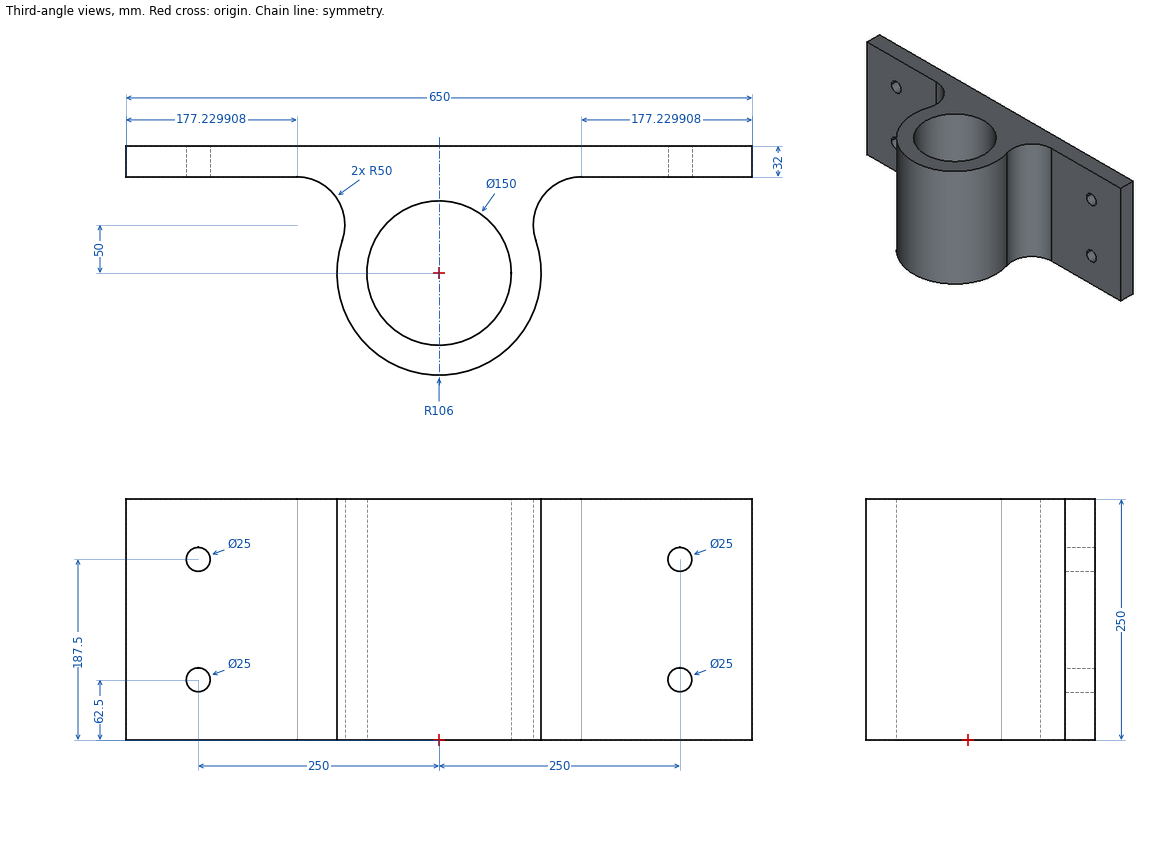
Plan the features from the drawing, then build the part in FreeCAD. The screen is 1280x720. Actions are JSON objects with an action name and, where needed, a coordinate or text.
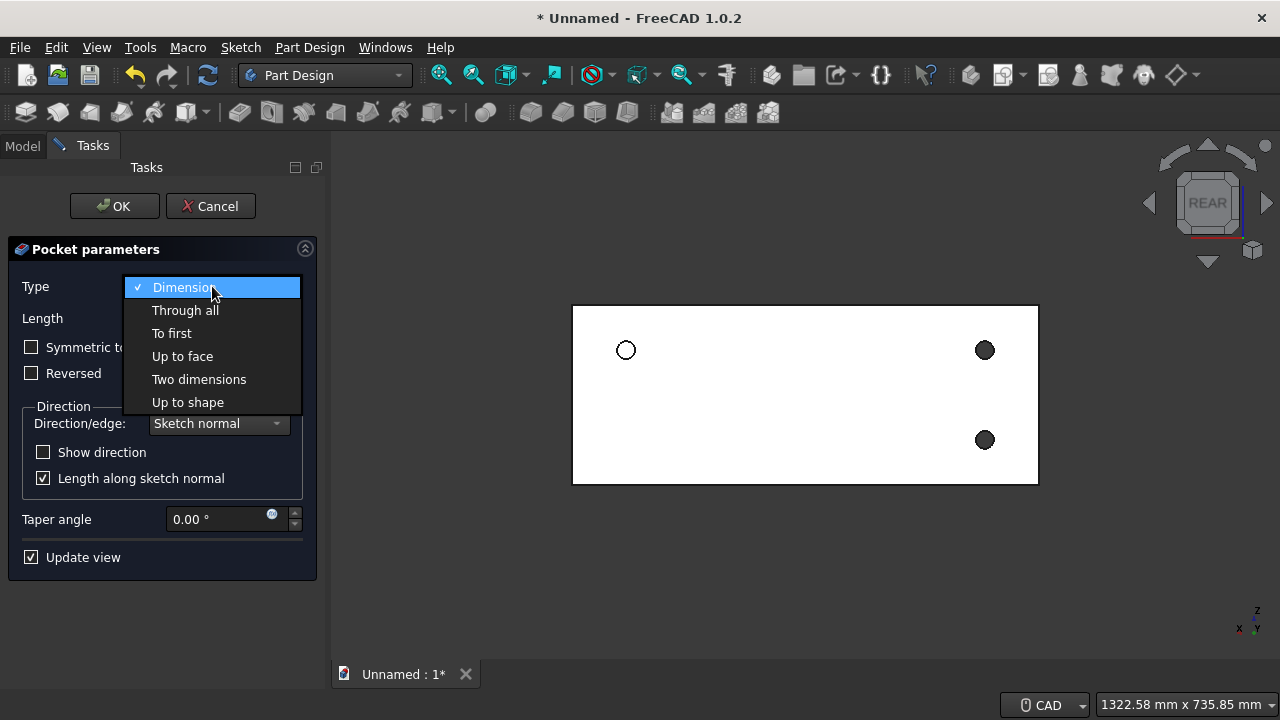
{"action": "left_click", "coordinate": [212, 334]}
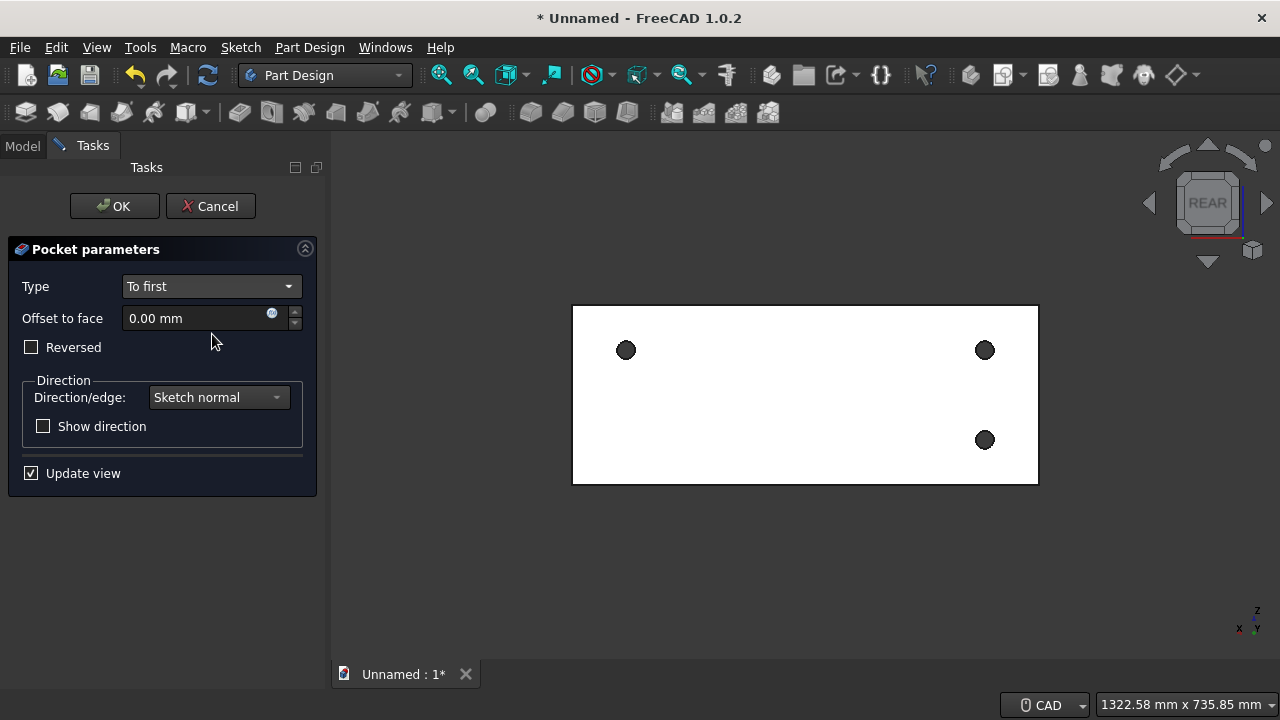
{"action": "left_click", "coordinate": [115, 206]}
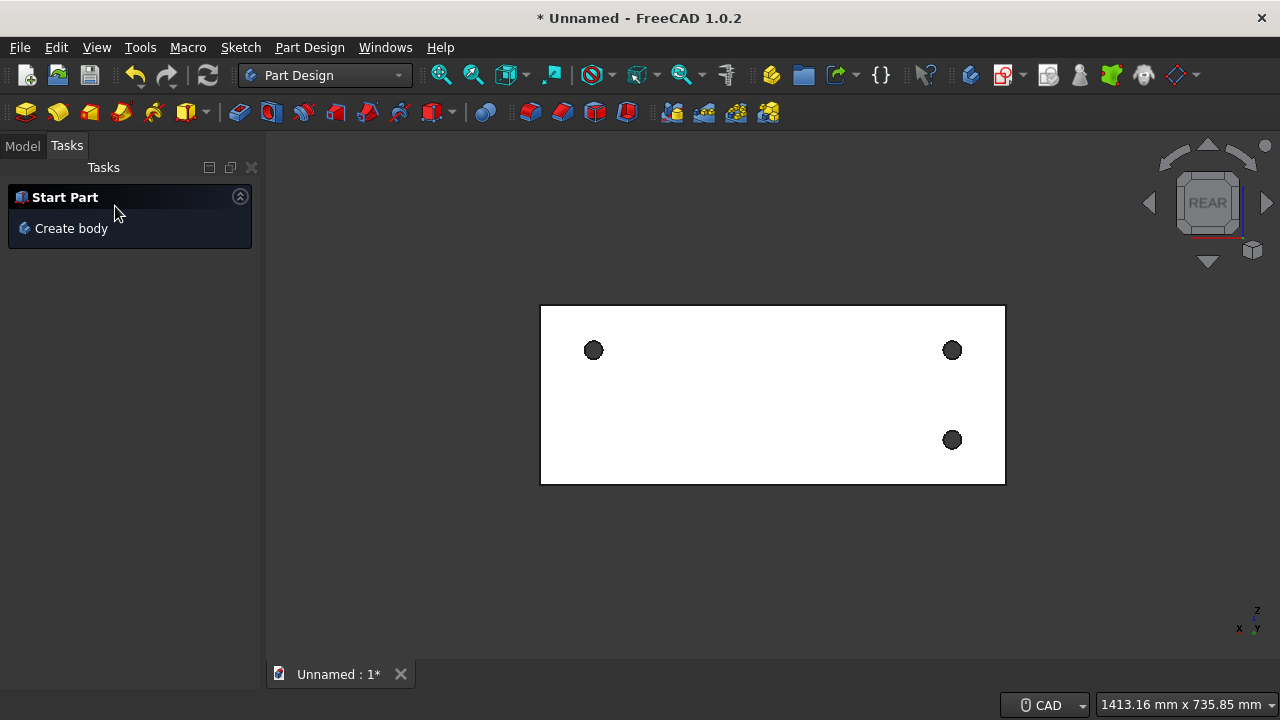
{"action": "left_click", "coordinate": [706, 394]}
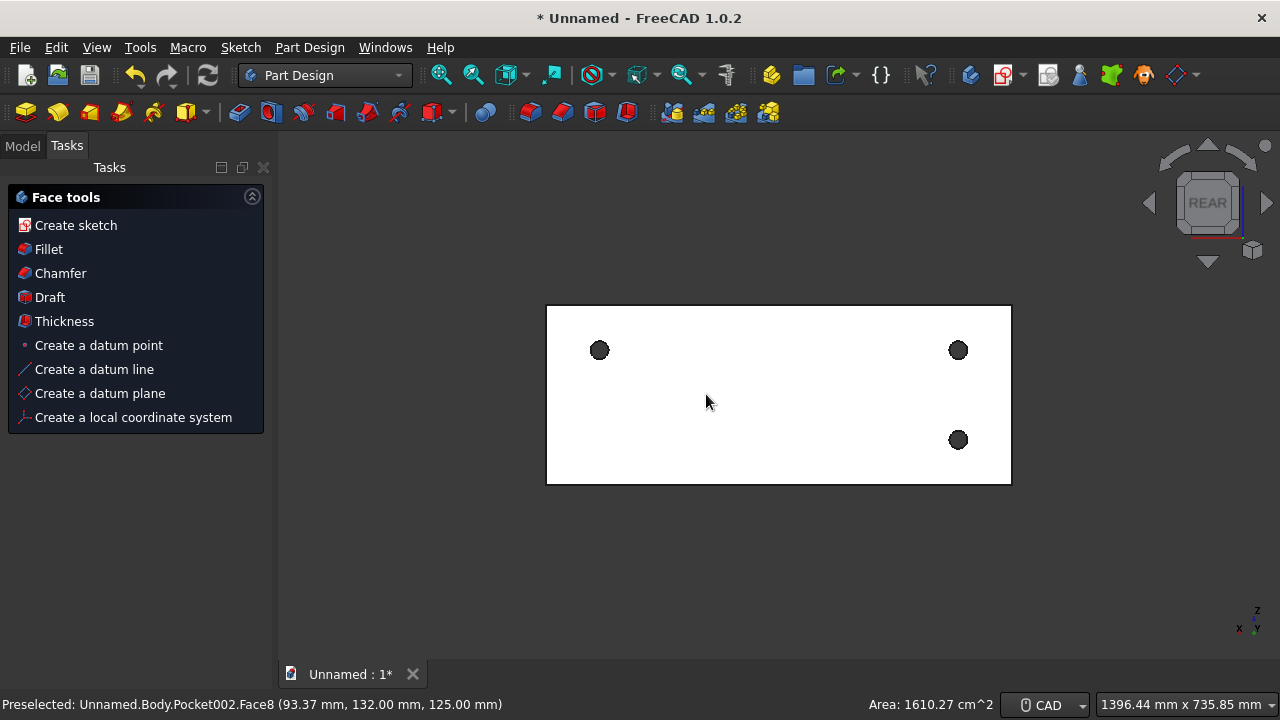
{"action": "left_click", "coordinate": [1004, 76]}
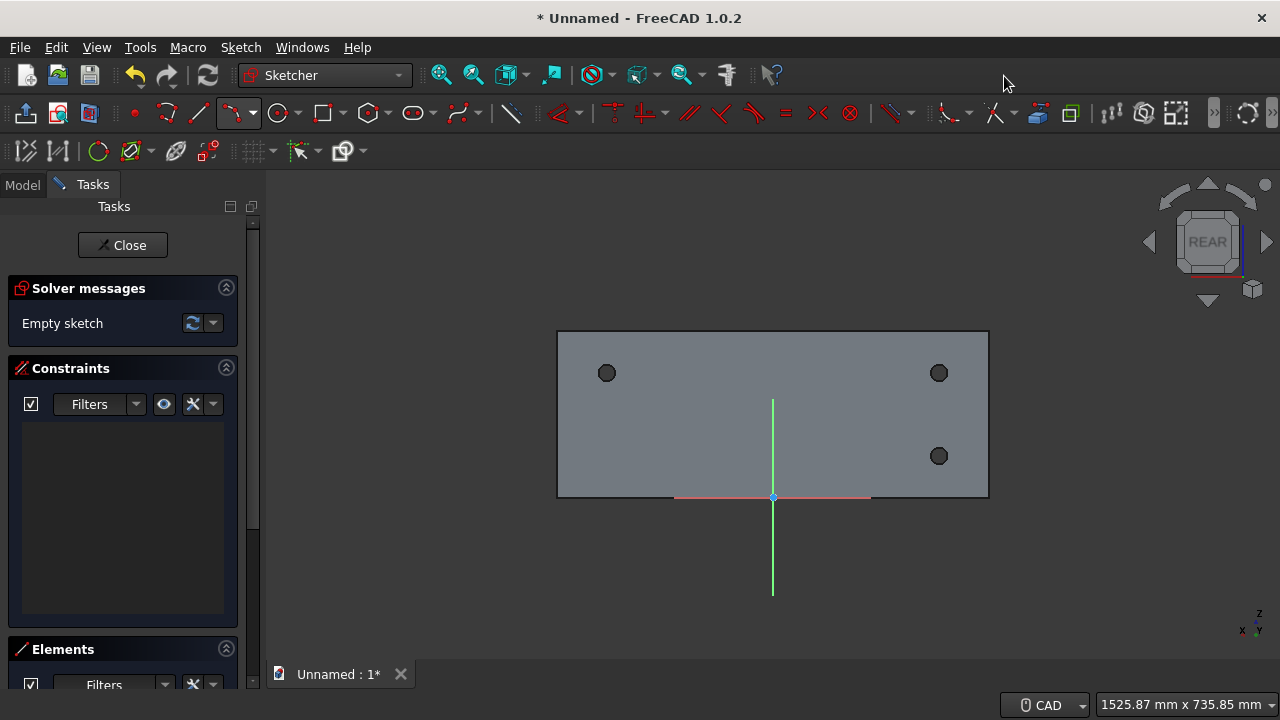
{"action": "scroll", "coordinate": [602, 458], "scroll_direction": "up", "scroll_amount": 15}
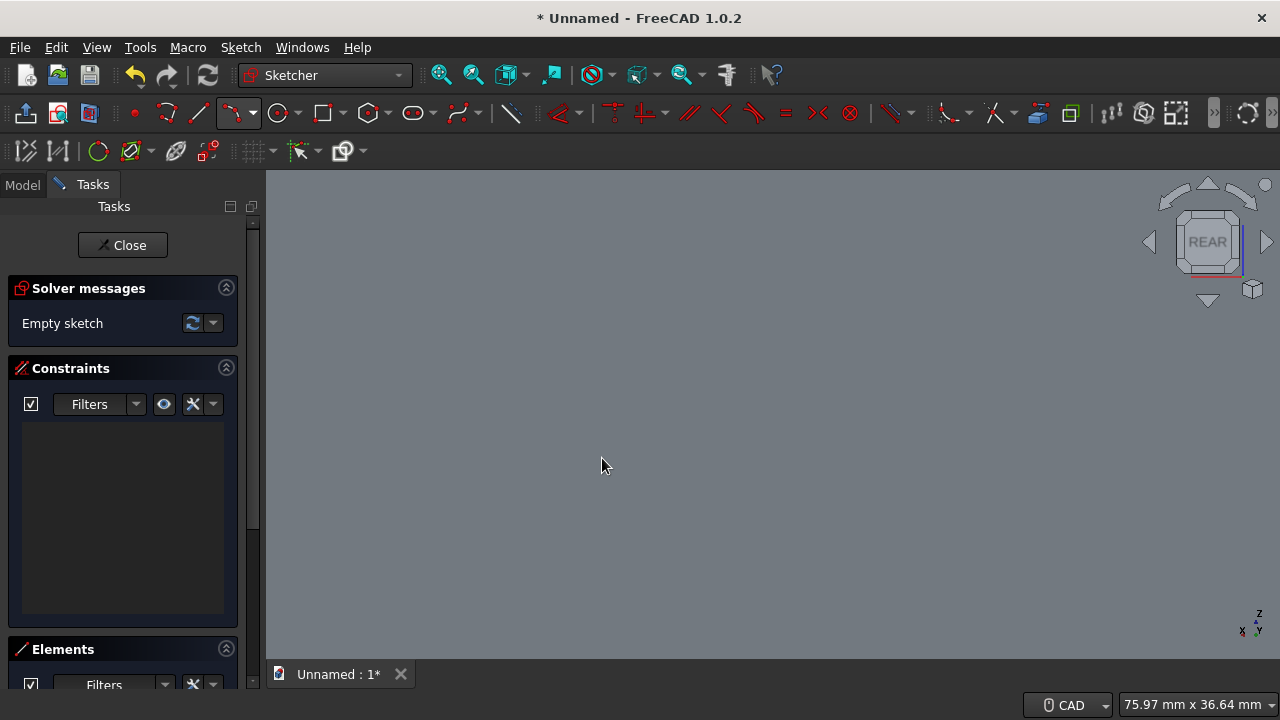
{"action": "left_click", "coordinate": [278, 114]}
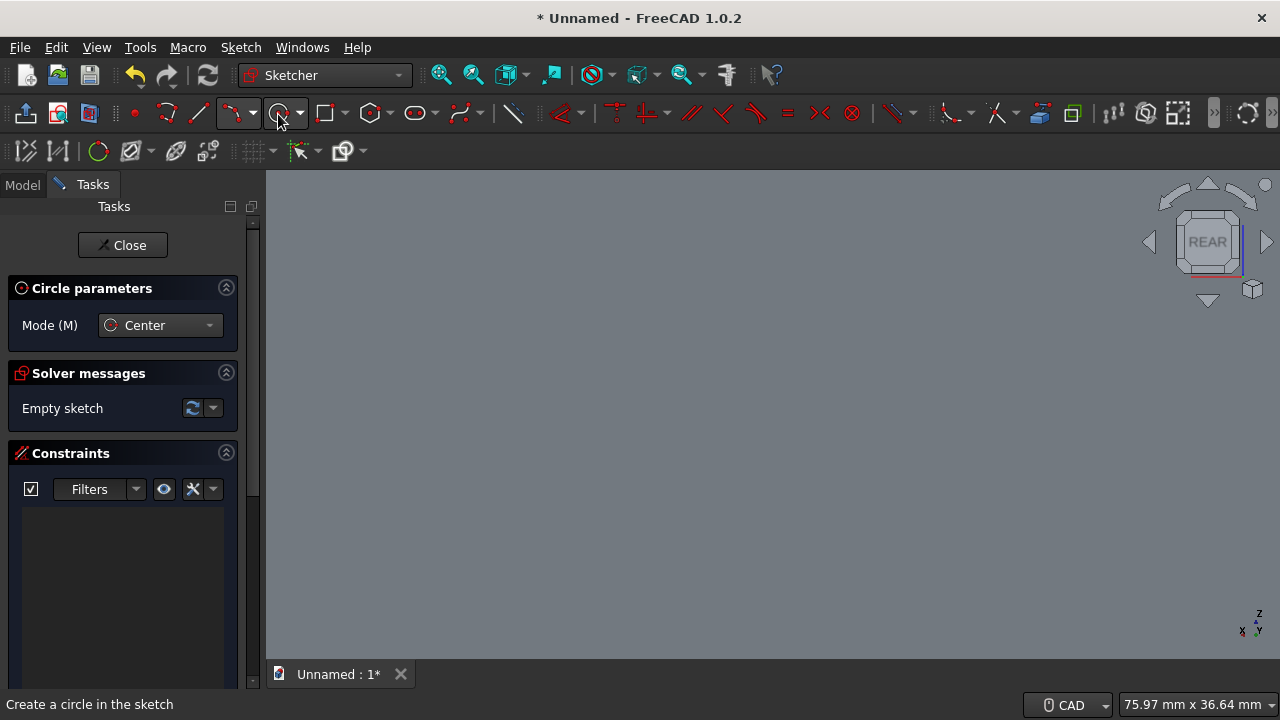
{"action": "left_click", "coordinate": [693, 407]}
{"action": "mouse_move", "coordinate": [811, 289]}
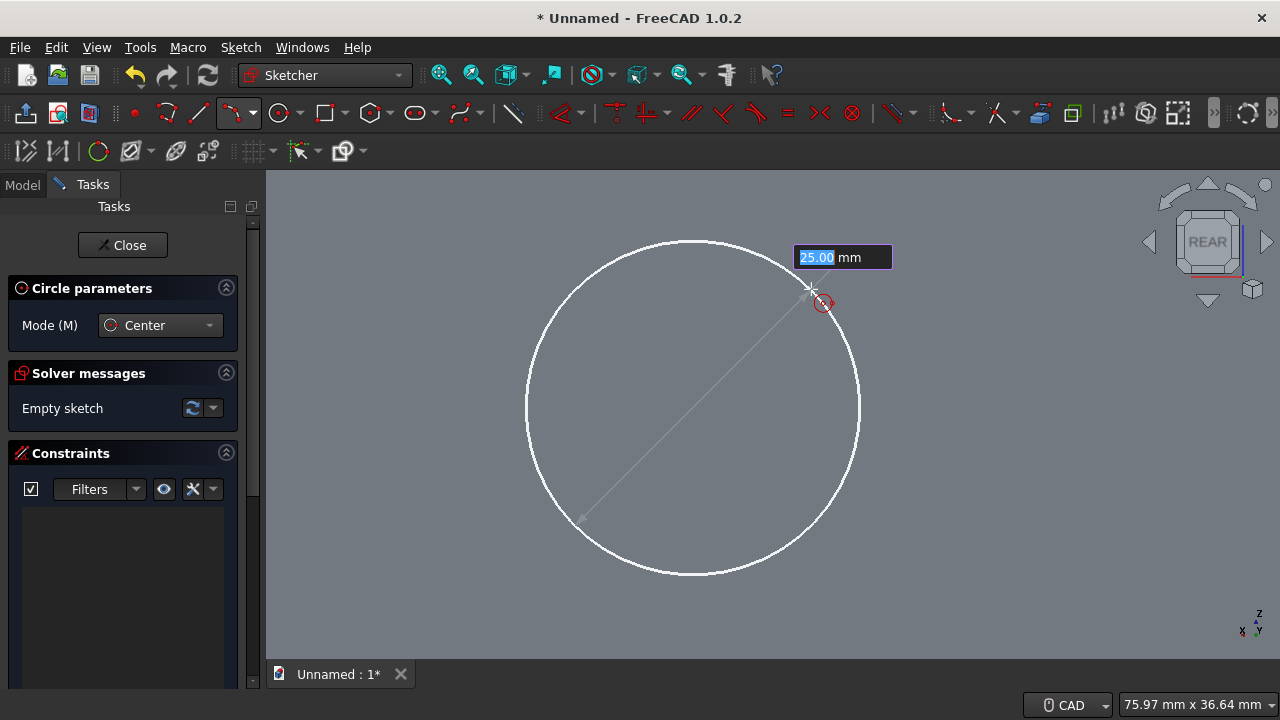
{"action": "type", "text": "25"}
{"action": "key", "text": "Return"}
{"action": "key", "text": "Escape"}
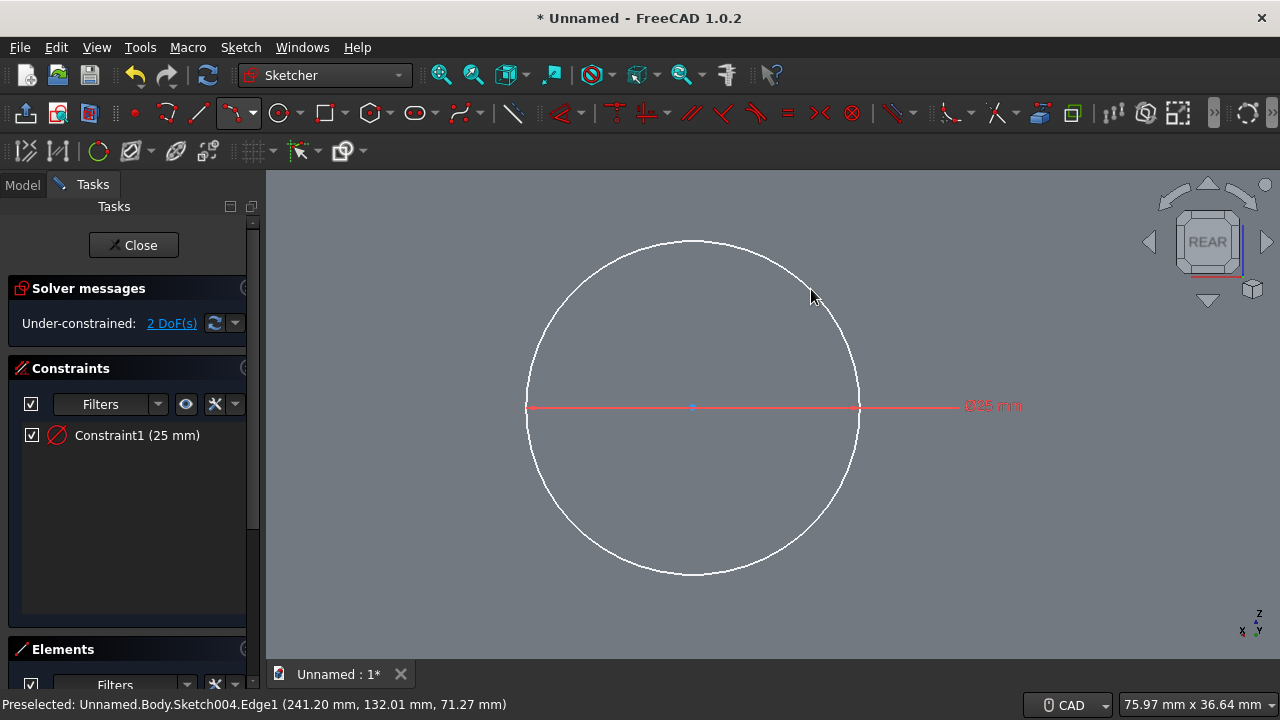
{"action": "left_click", "coordinate": [560, 114]}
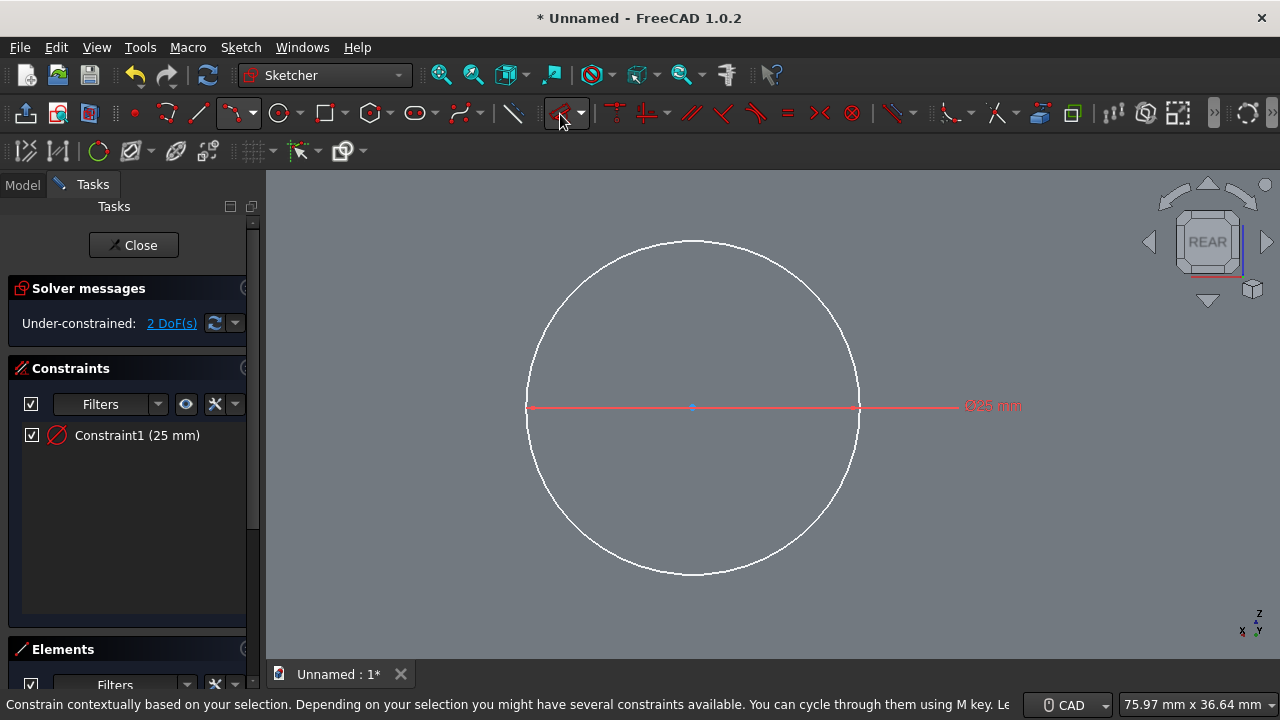
{"action": "left_click", "coordinate": [693, 408]}
{"action": "left_click", "coordinate": [904, 374]}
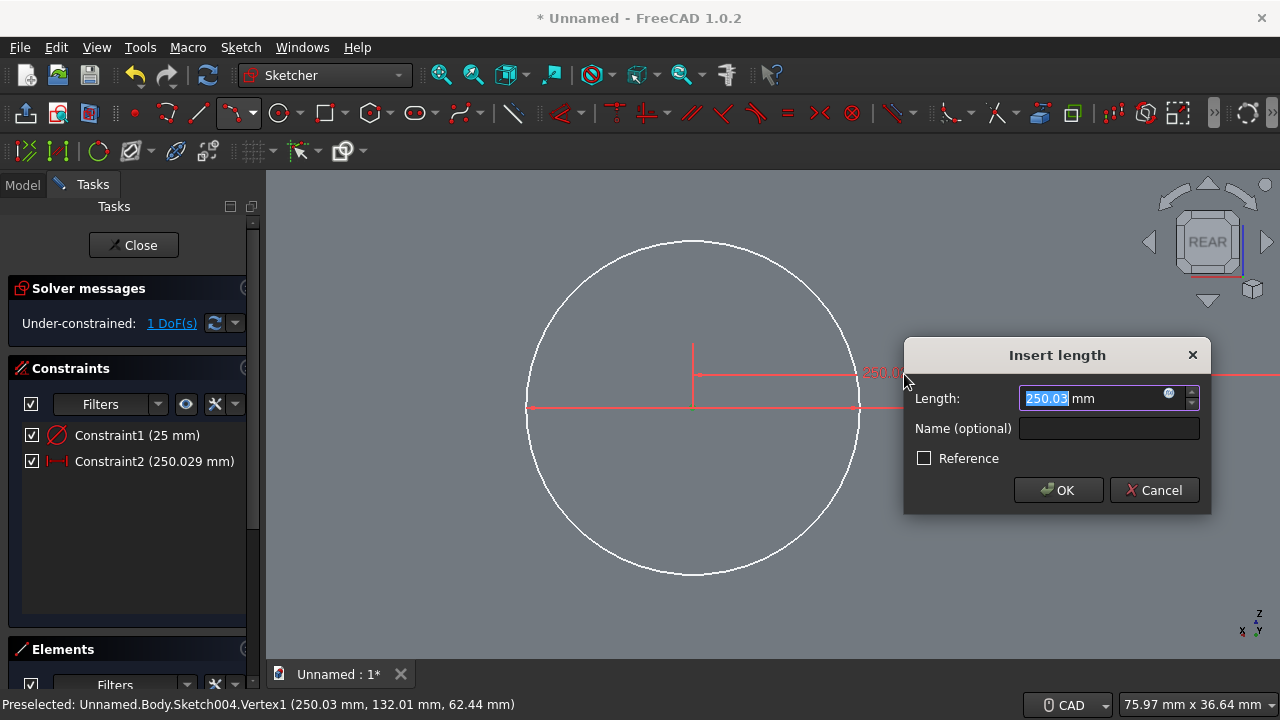
{"action": "type", "text": "250"}
{"action": "key", "text": "Return"}